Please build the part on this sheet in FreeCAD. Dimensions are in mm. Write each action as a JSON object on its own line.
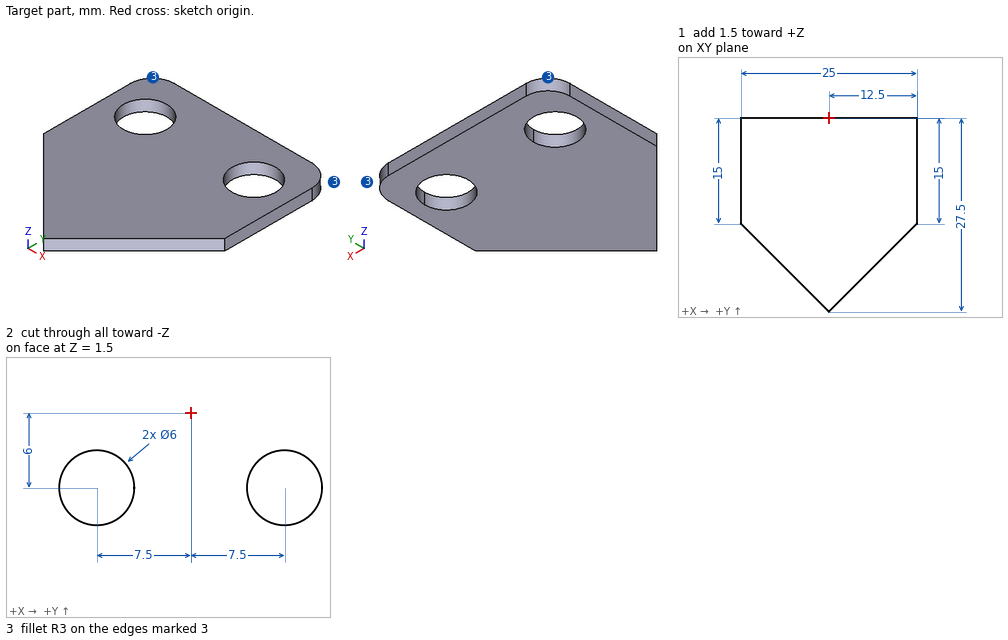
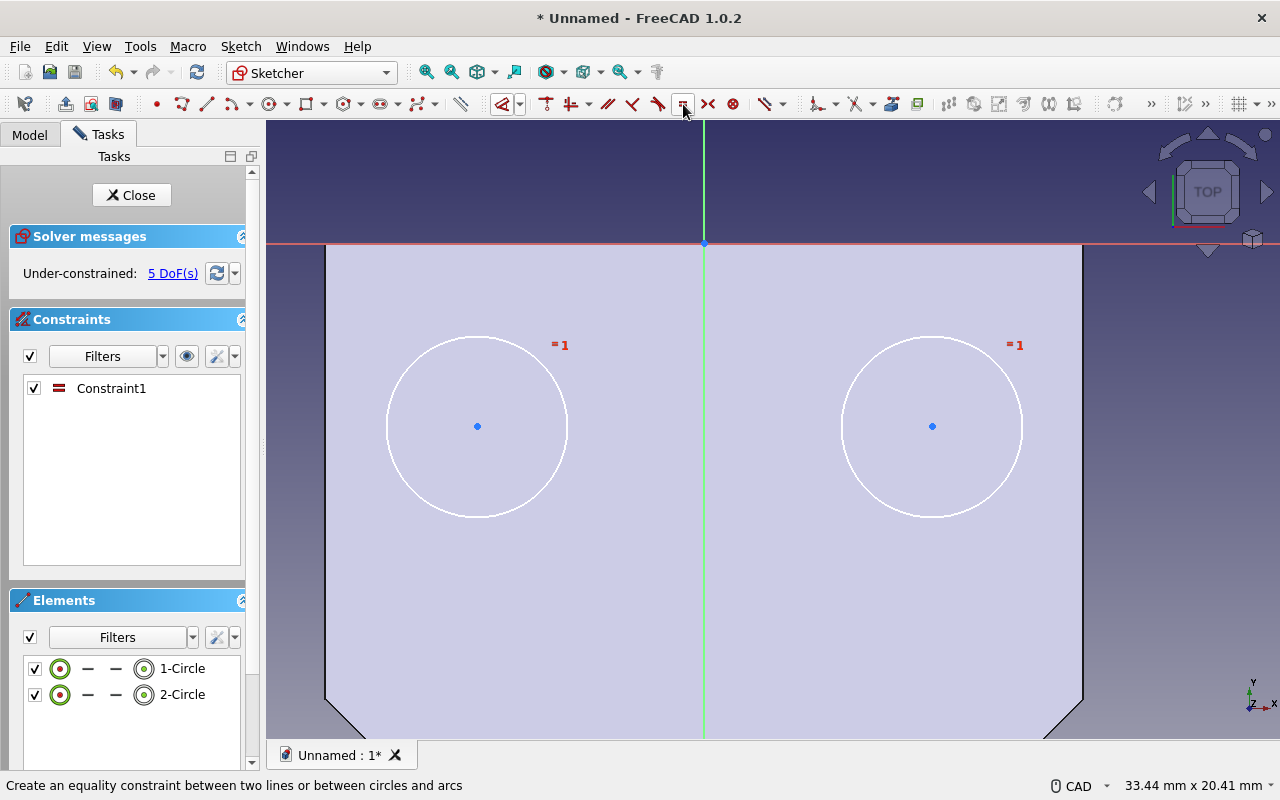
{"action": "left_click", "coordinate": [477, 427]}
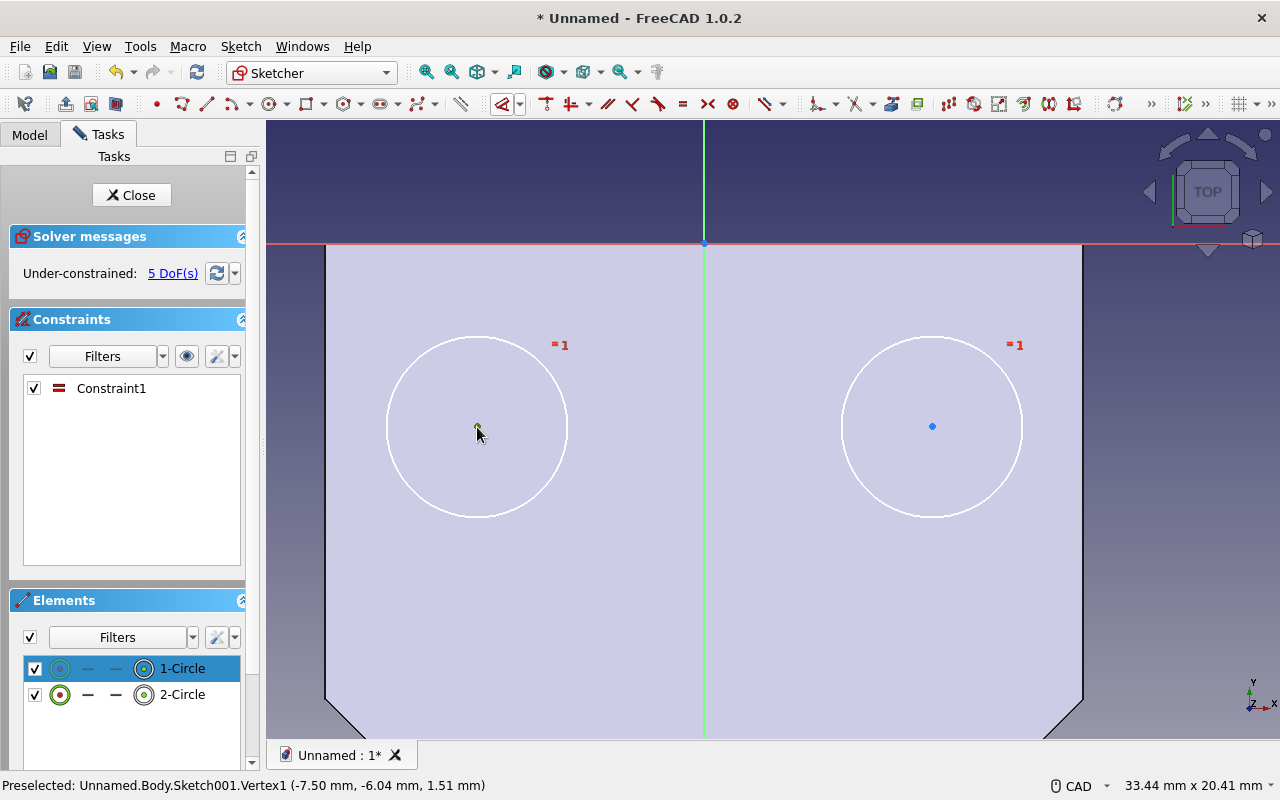
{"action": "left_click", "coordinate": [932, 427]}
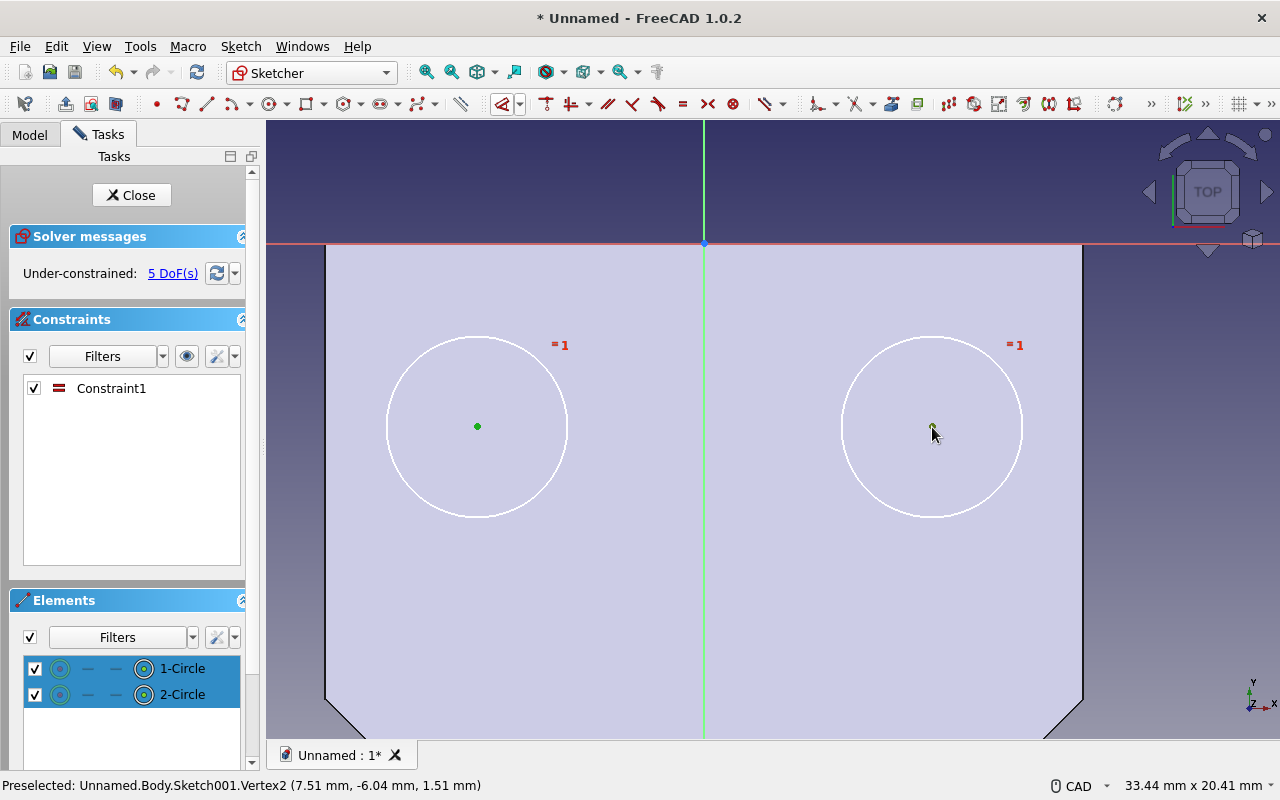
{"action": "left_click", "coordinate": [588, 104]}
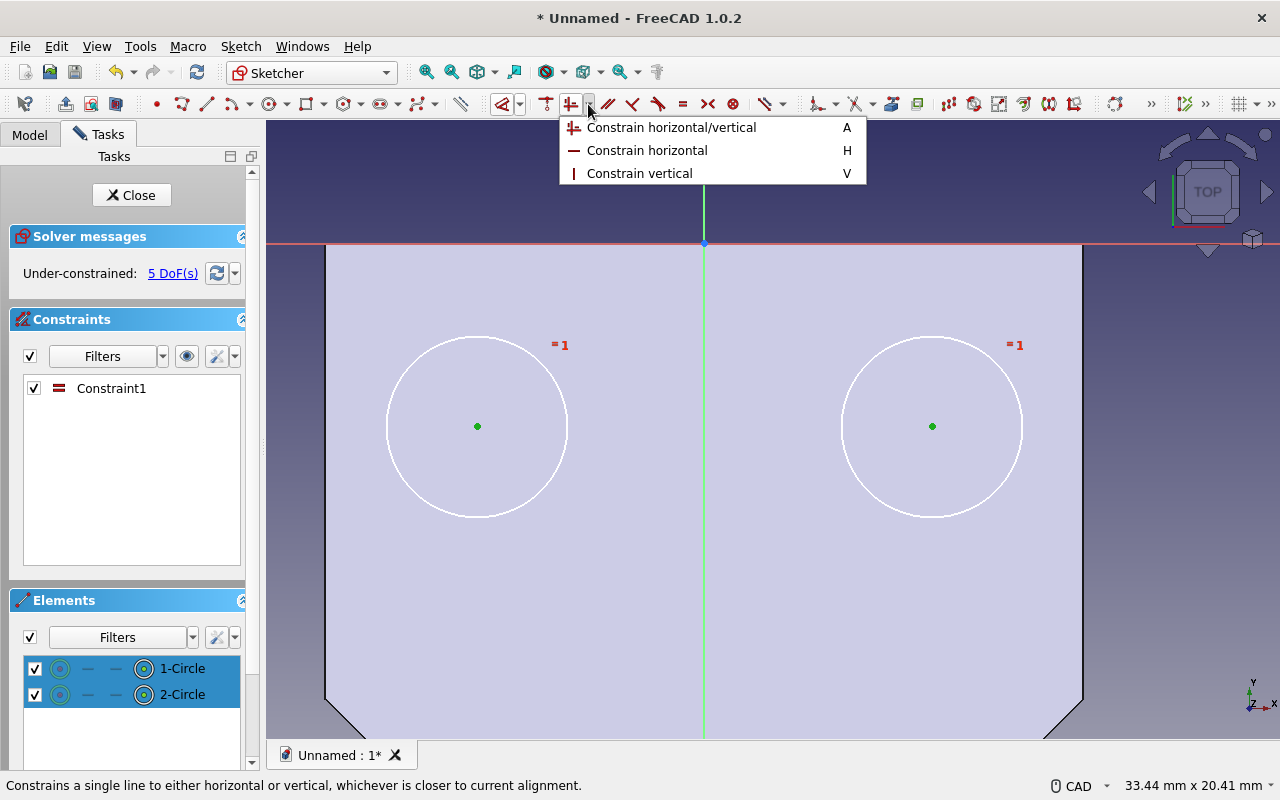
{"action": "left_click", "coordinate": [713, 150]}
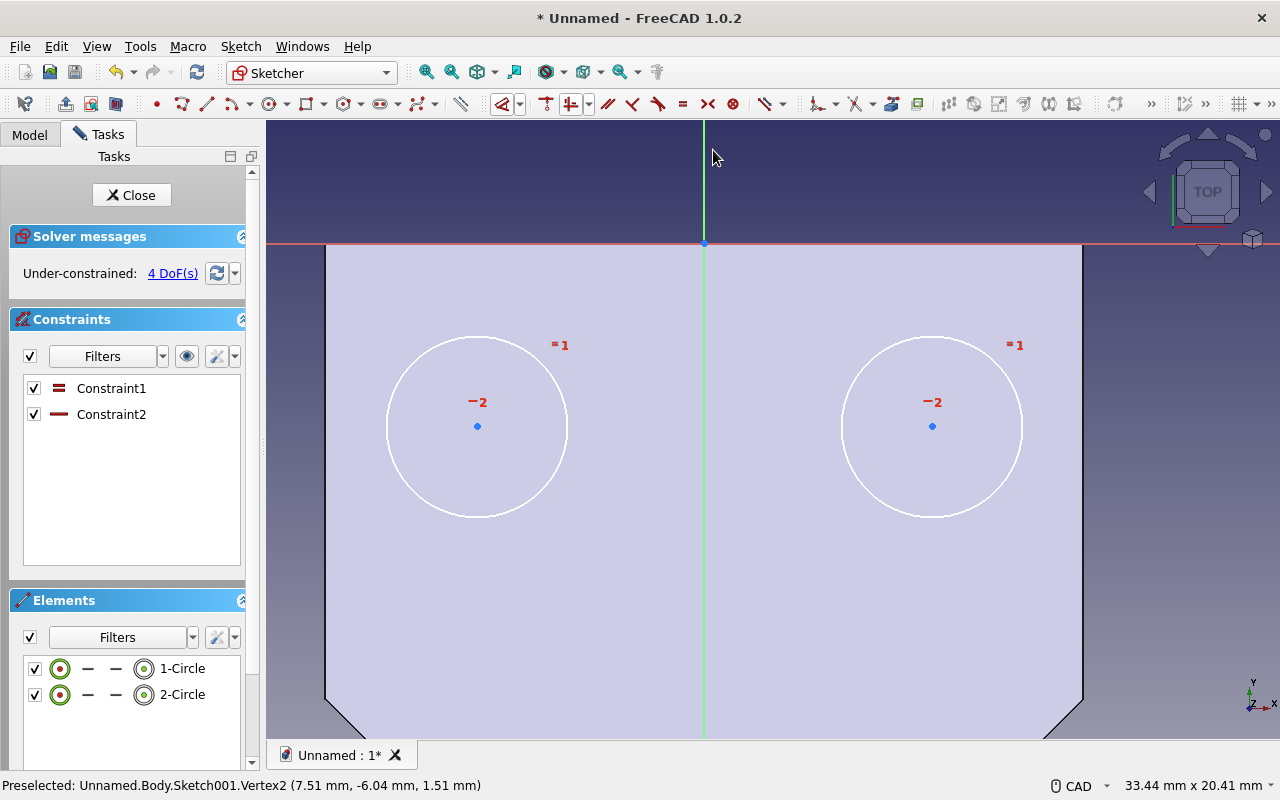
{"action": "left_click", "coordinate": [541, 363]}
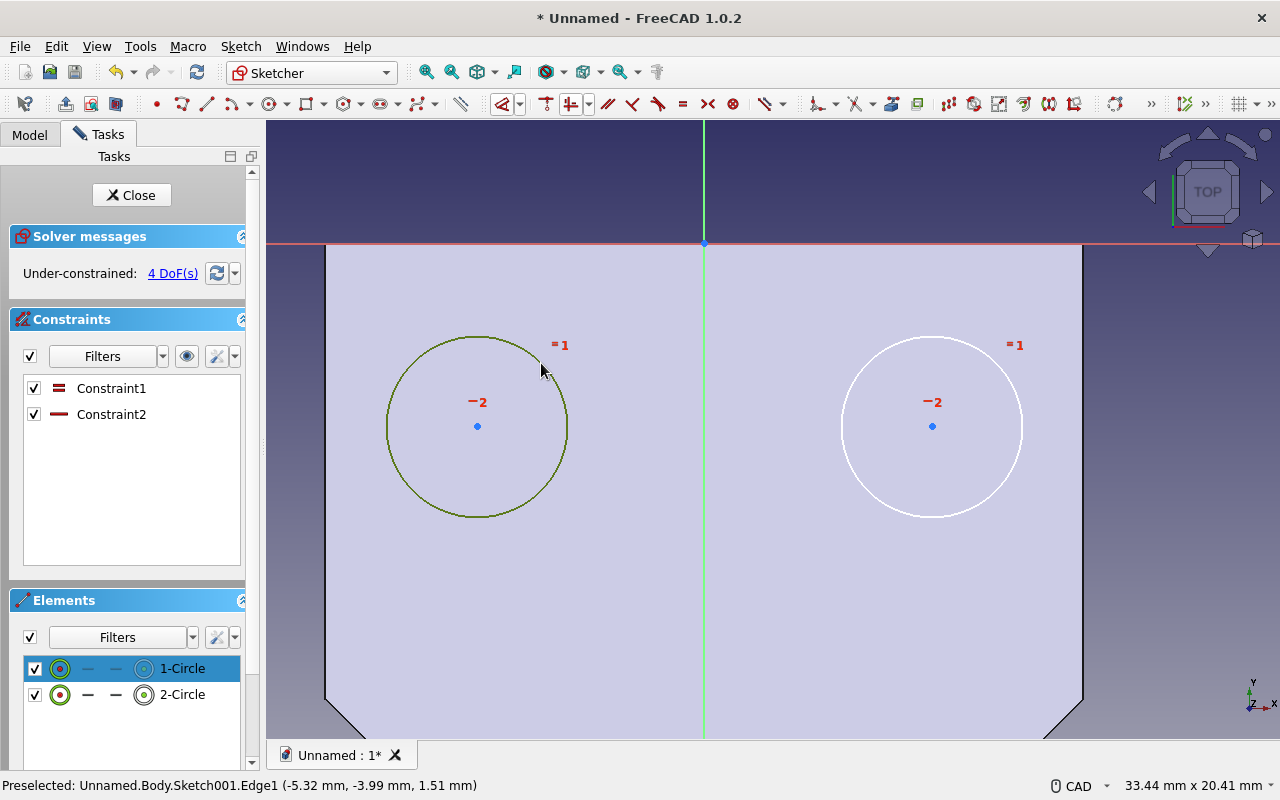
{"action": "left_click", "coordinate": [520, 104]}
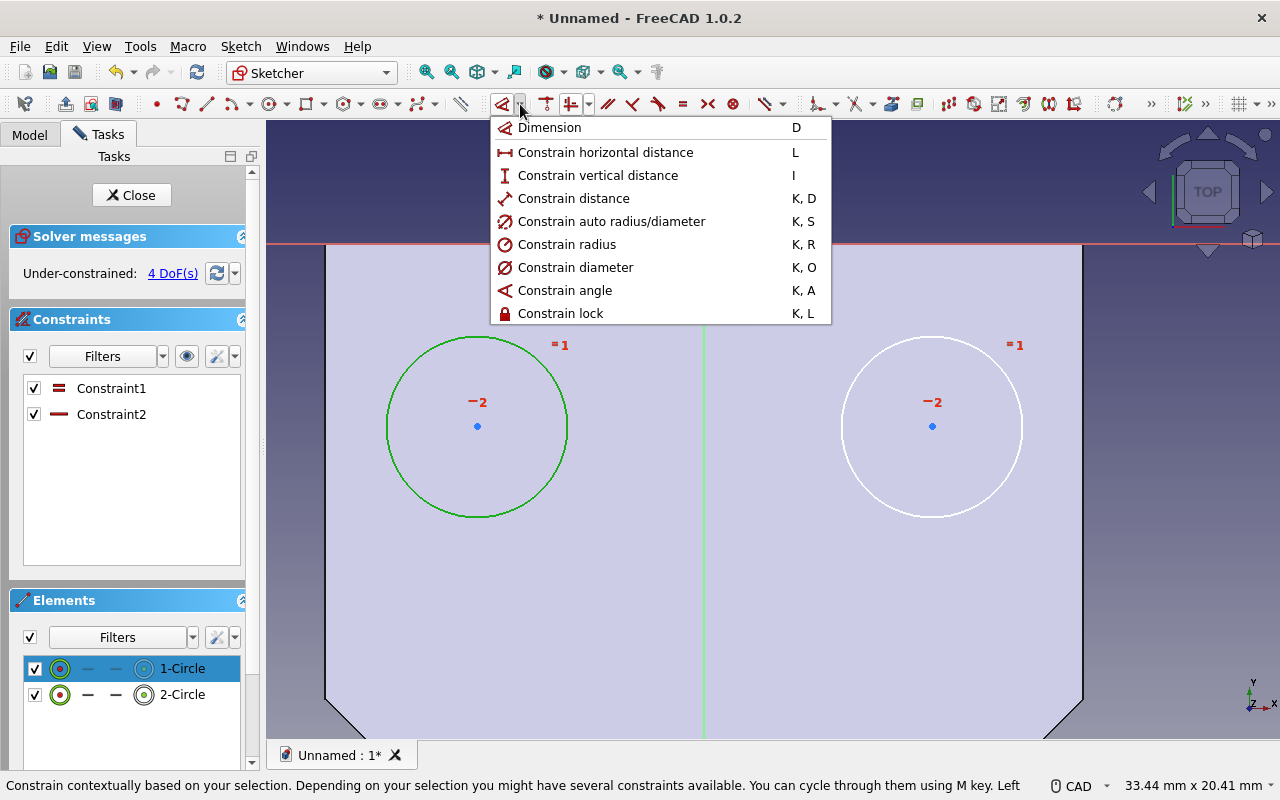
{"action": "left_click", "coordinate": [661, 268]}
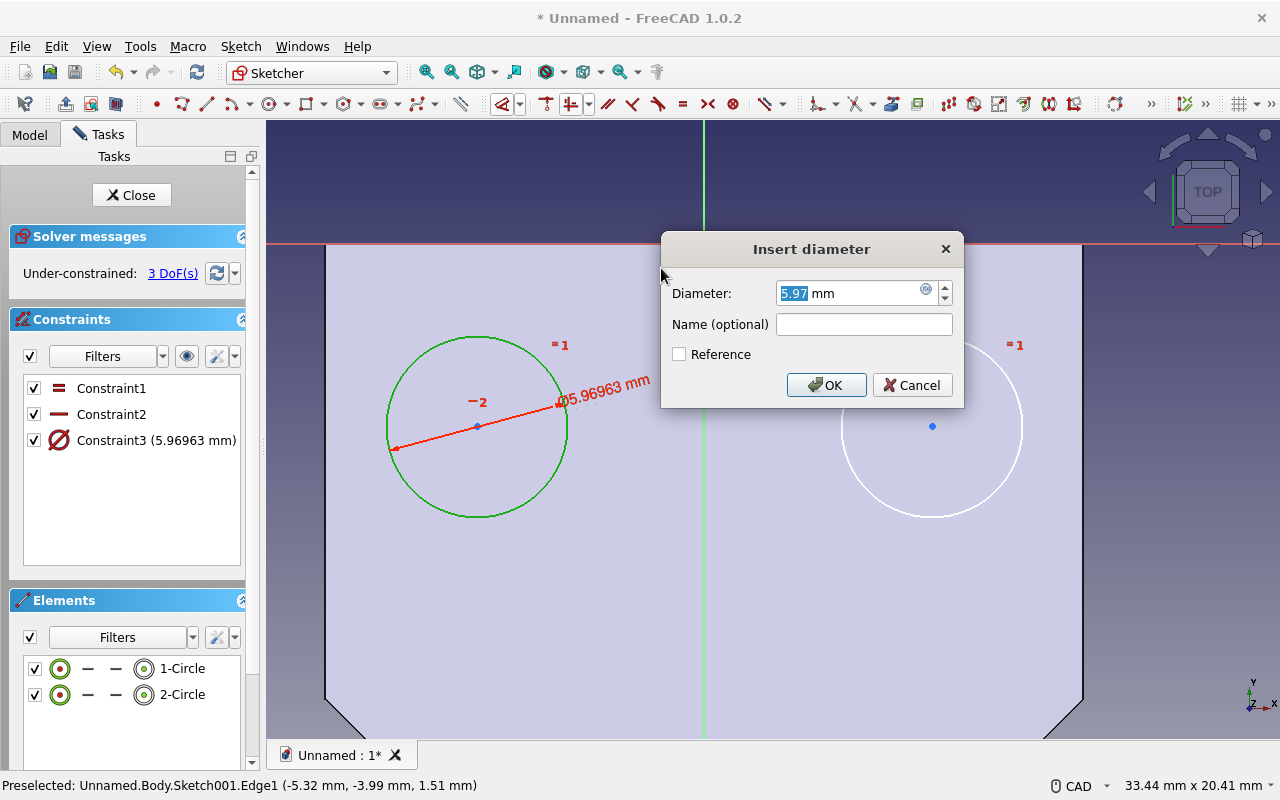
{"action": "type", "text": "6"}
{"action": "key", "text": "Return"}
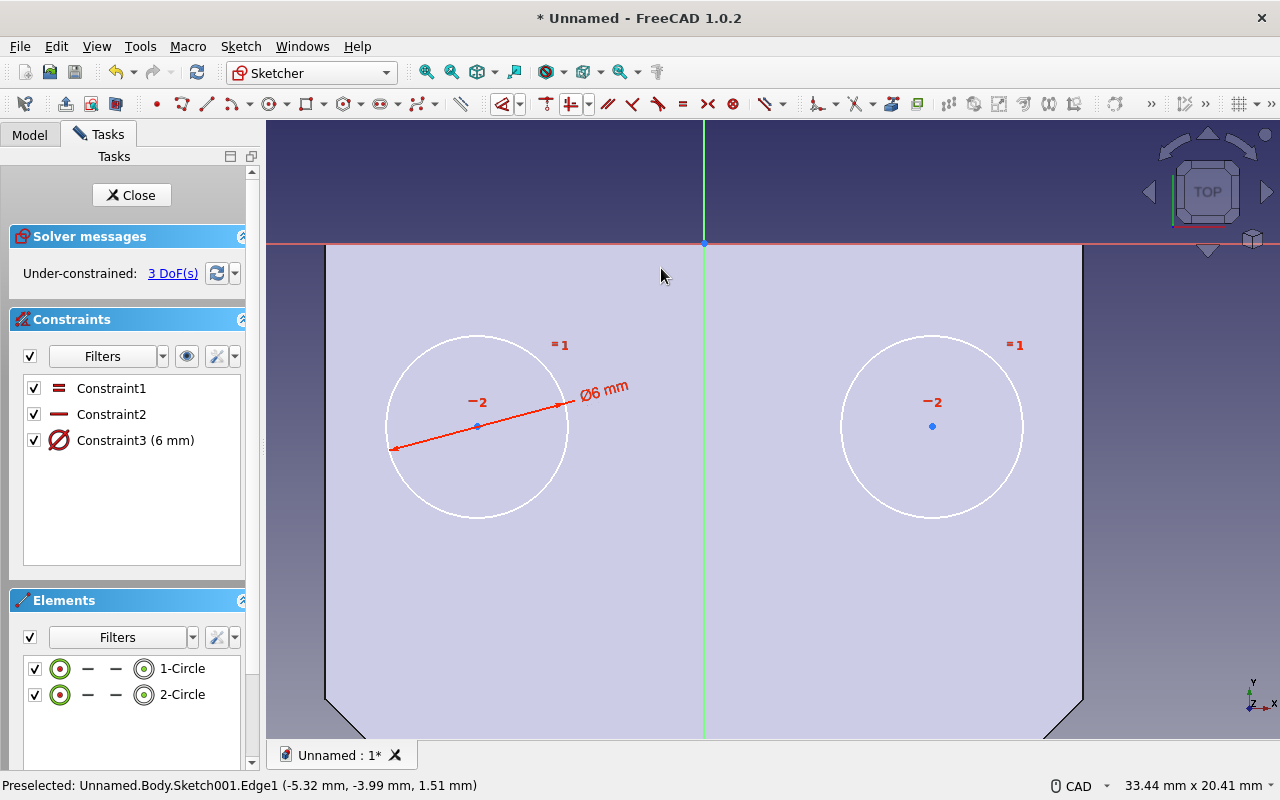
{"action": "left_click", "coordinate": [477, 427]}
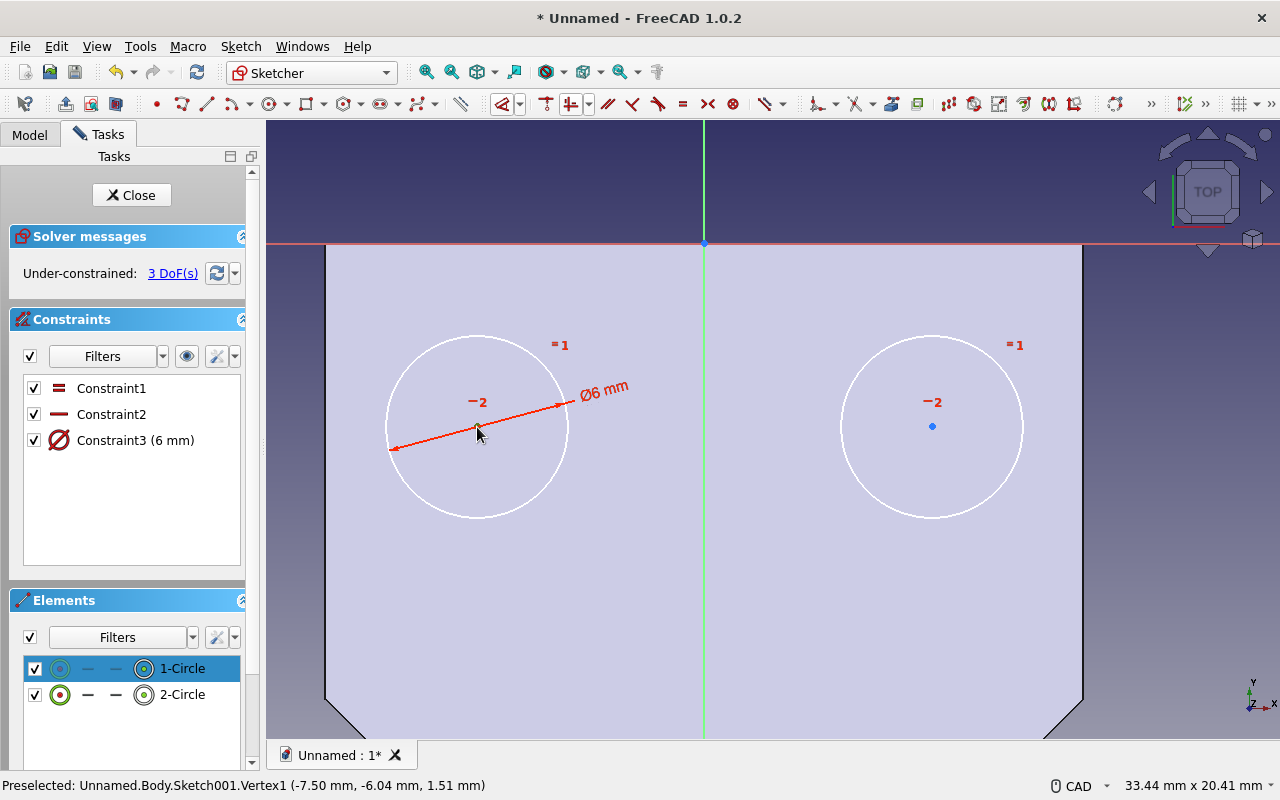
{"action": "left_click", "coordinate": [520, 104]}